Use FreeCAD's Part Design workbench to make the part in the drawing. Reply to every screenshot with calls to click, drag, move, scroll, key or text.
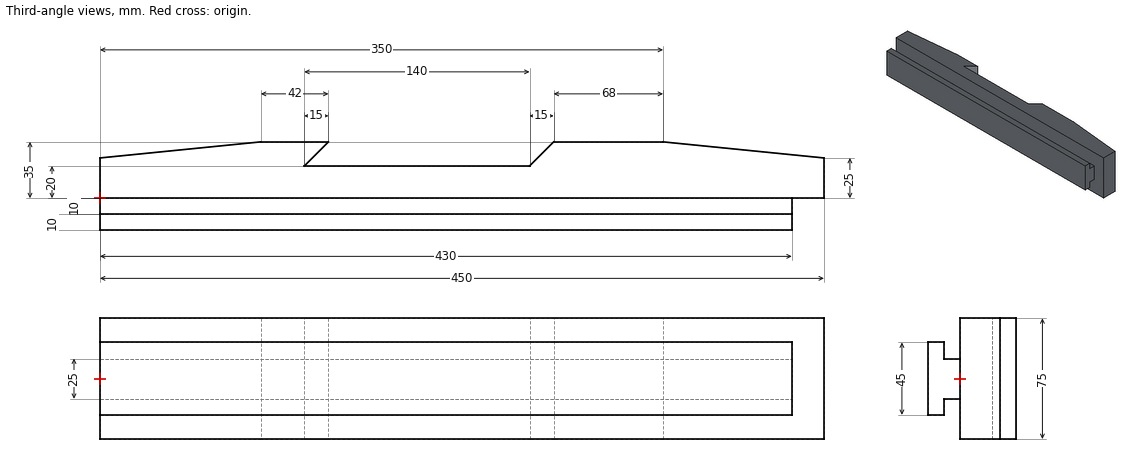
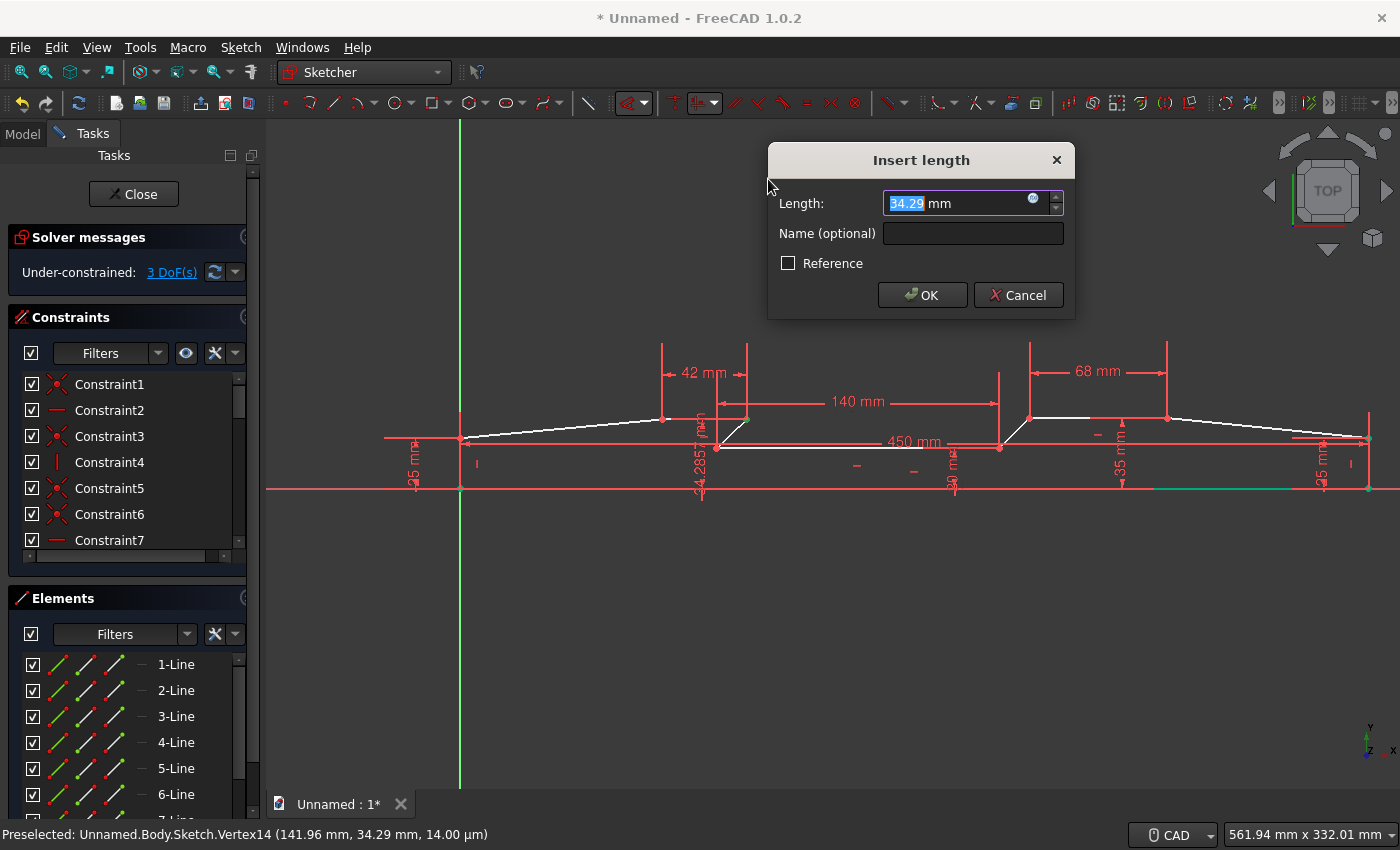
text(35)
key(Return)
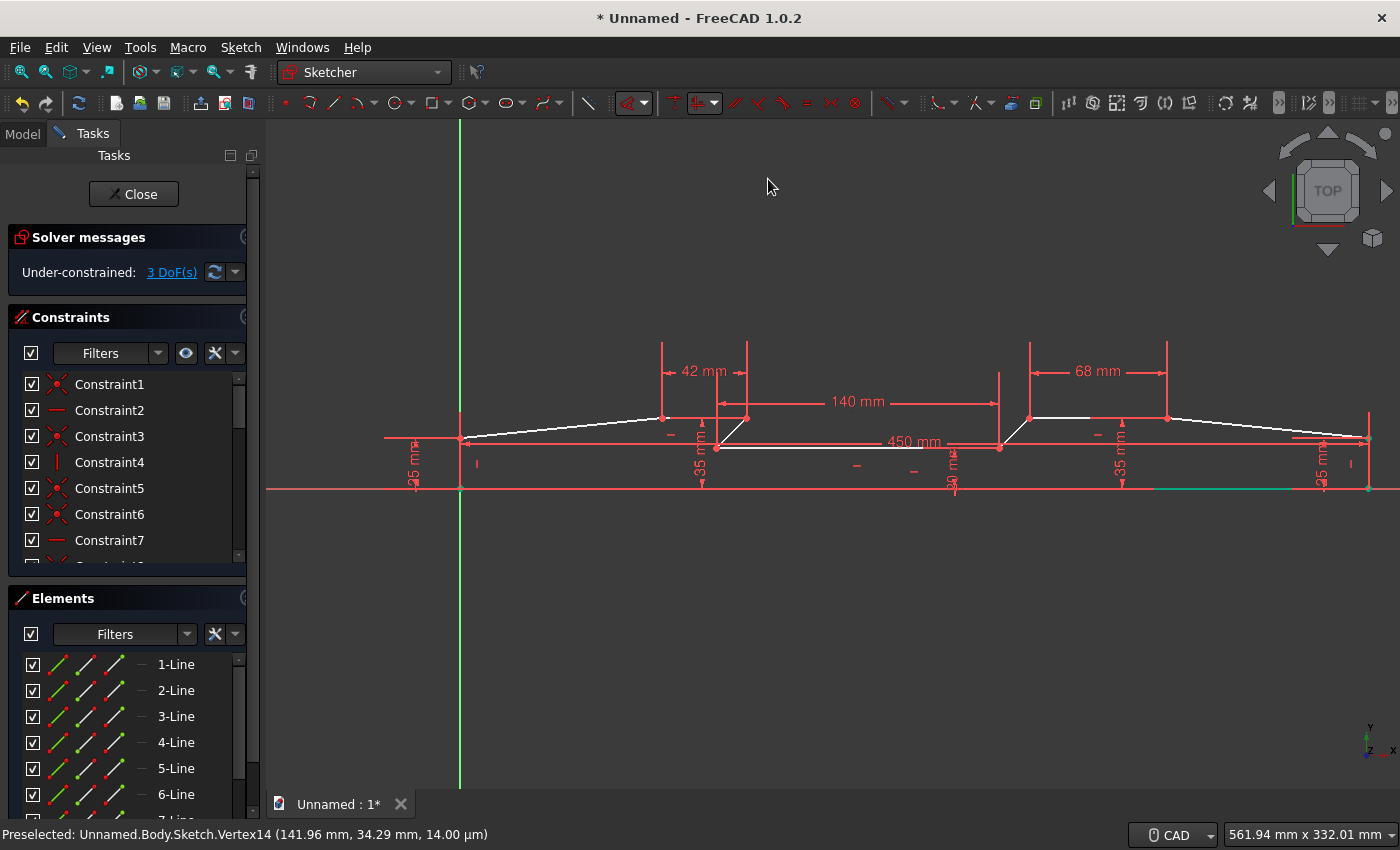
scroll(1021, 427, up, 2)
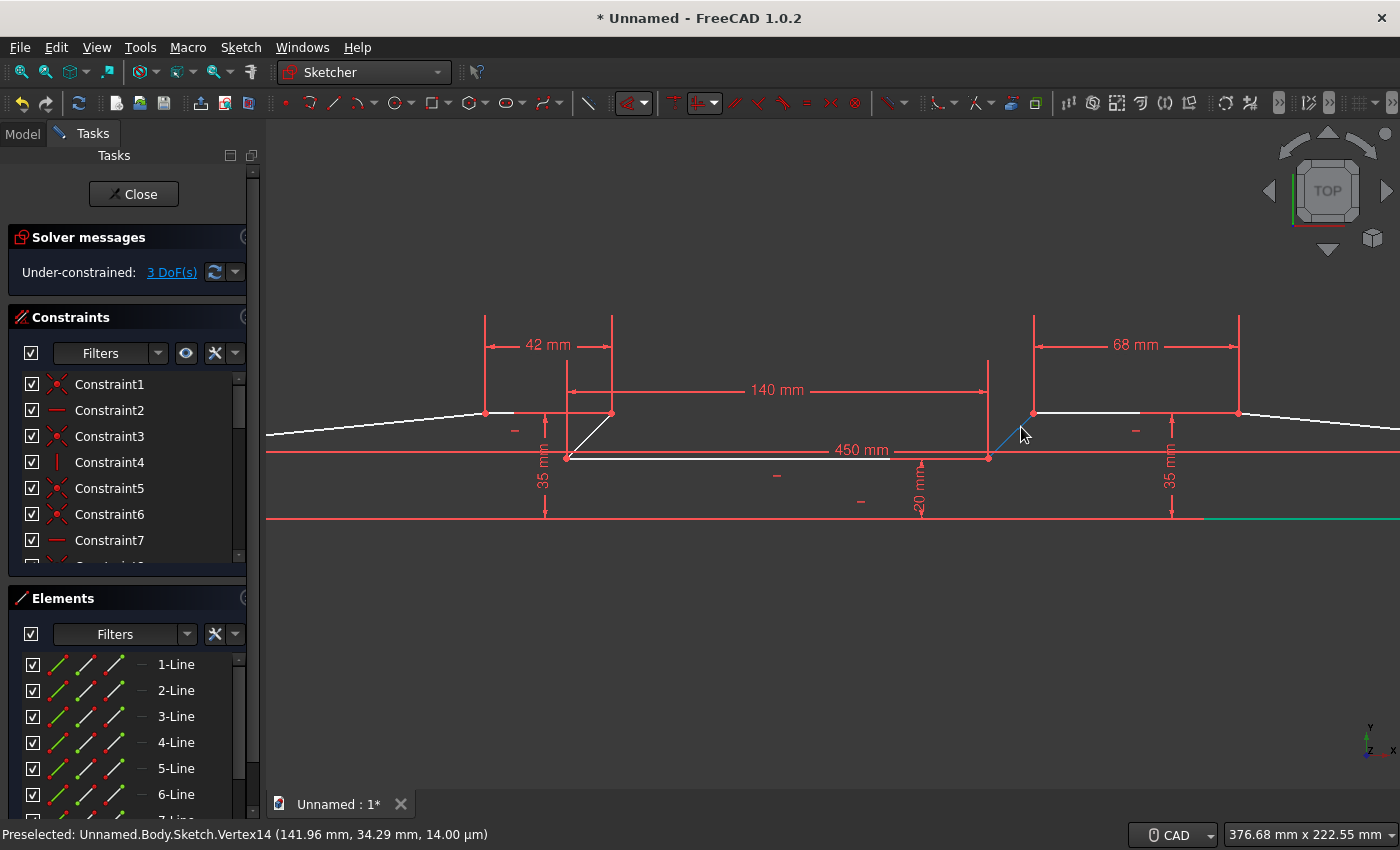
click(1020, 427)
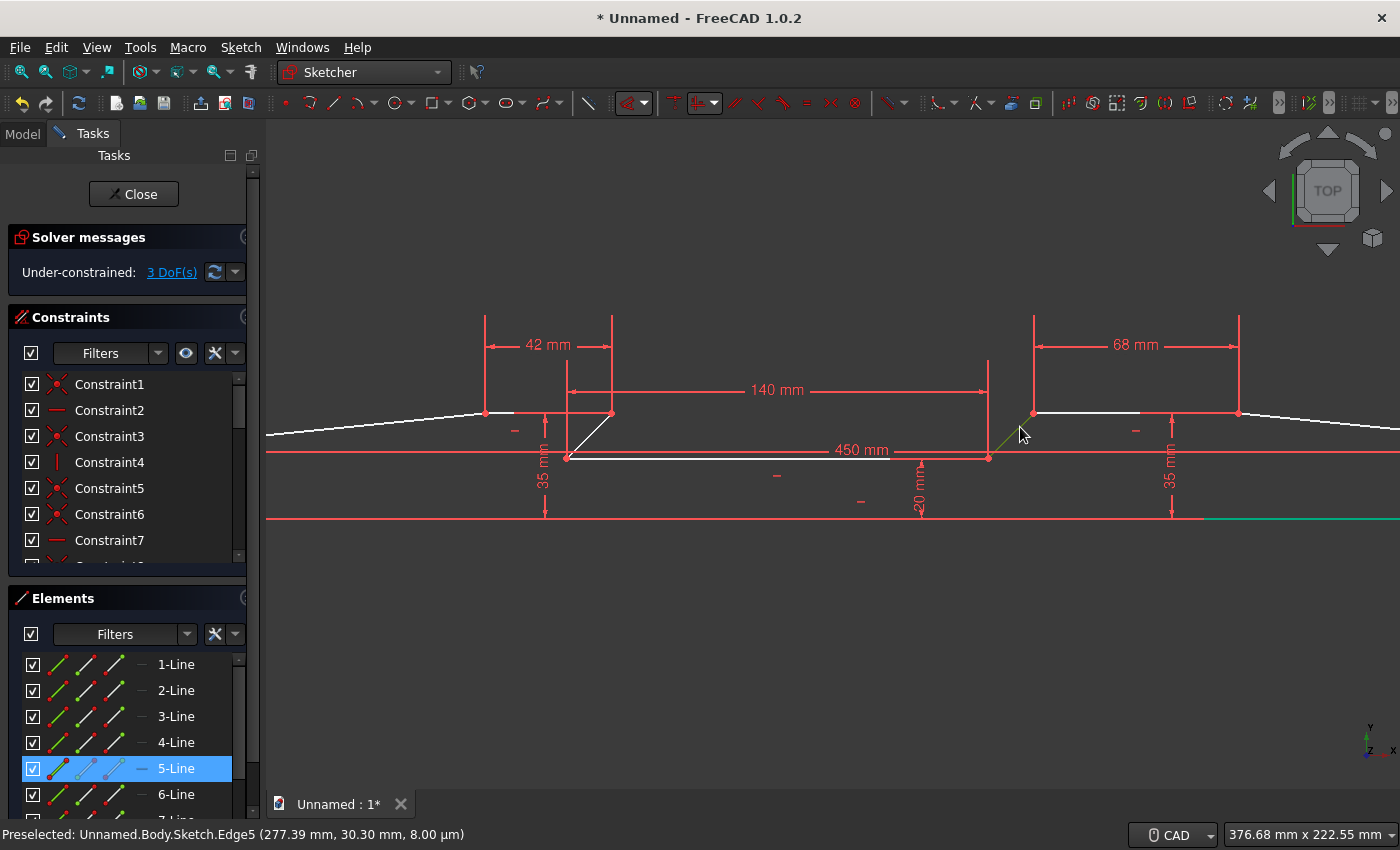
click(646, 104)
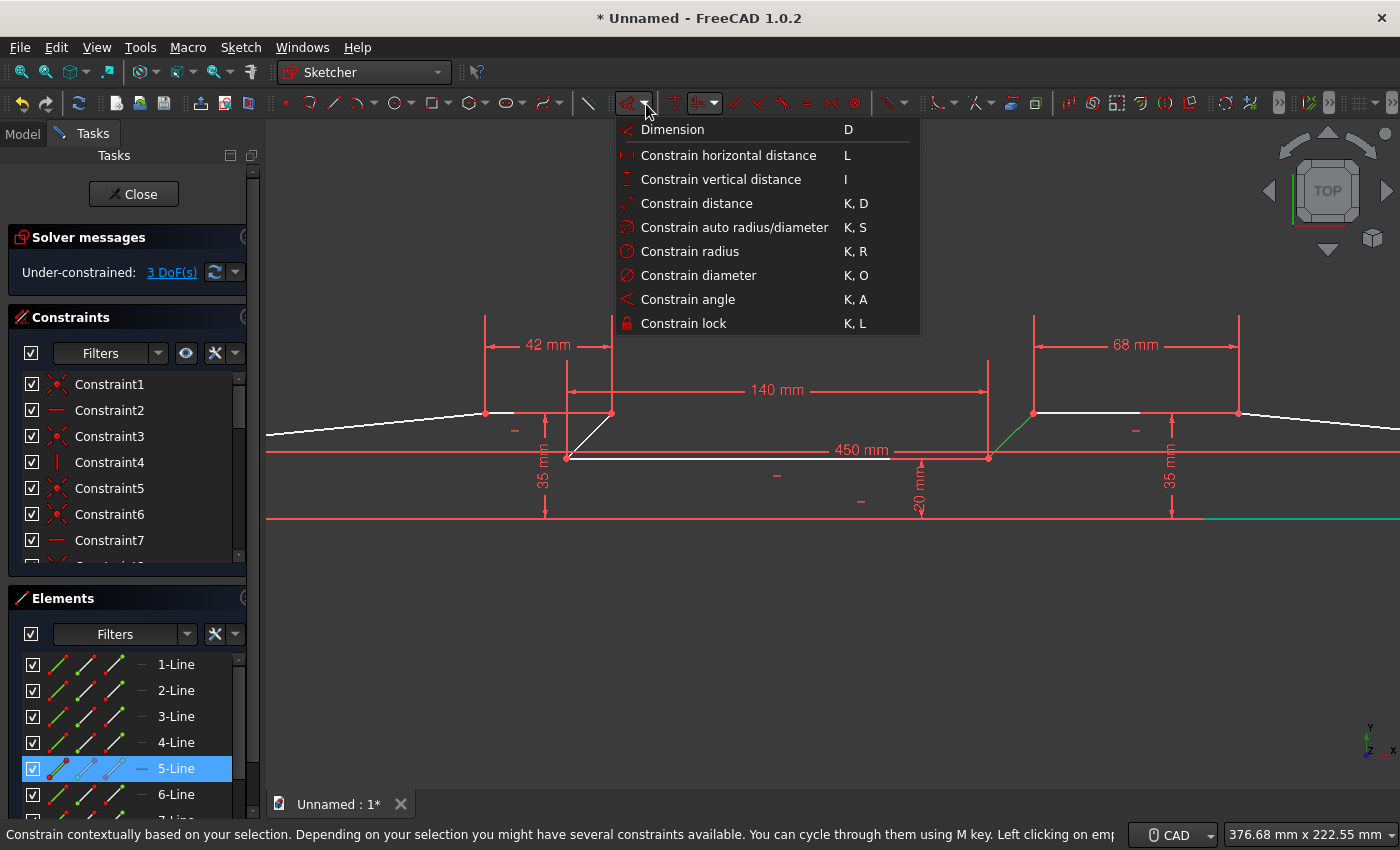
click(768, 155)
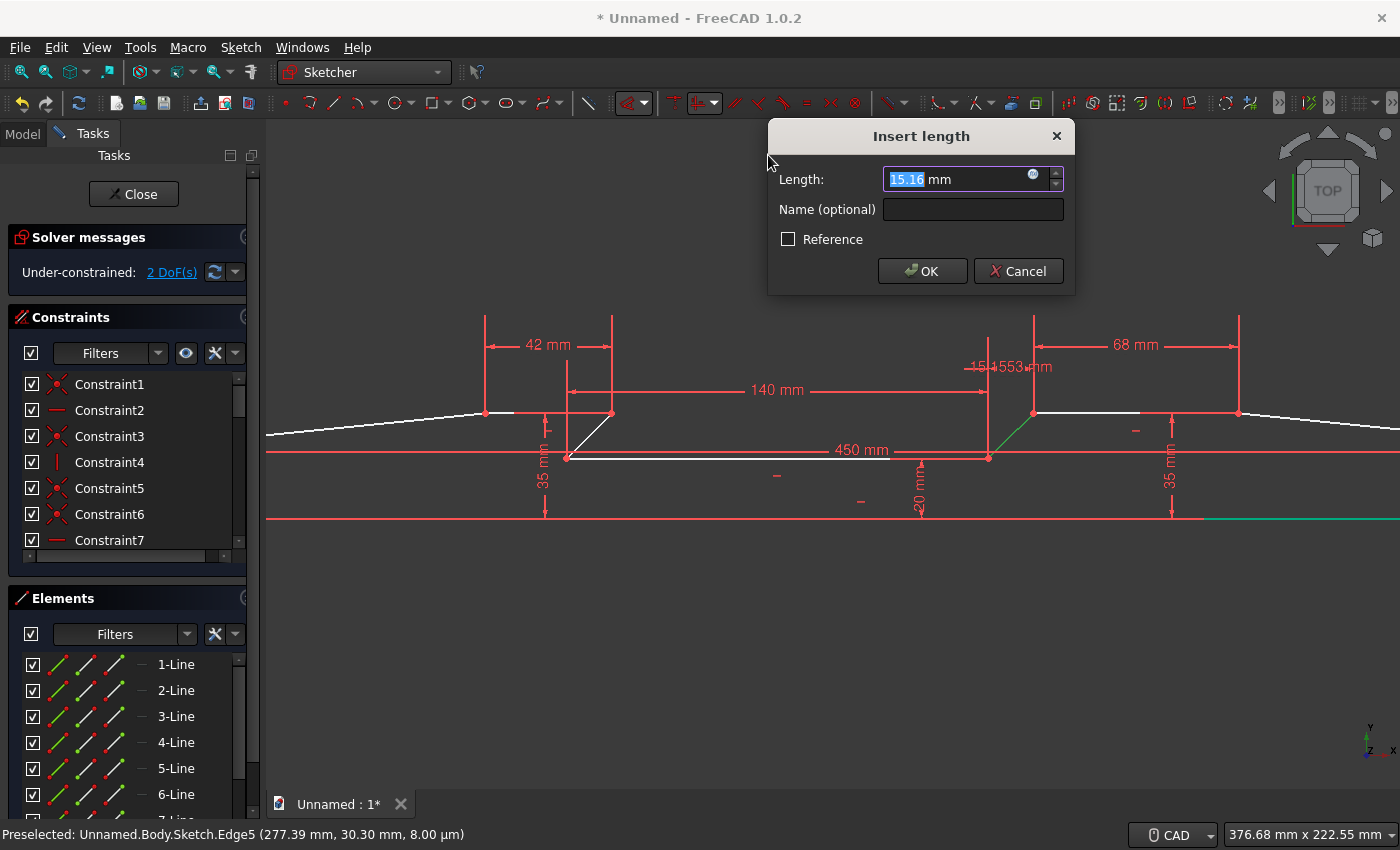
text(15)
key(Return)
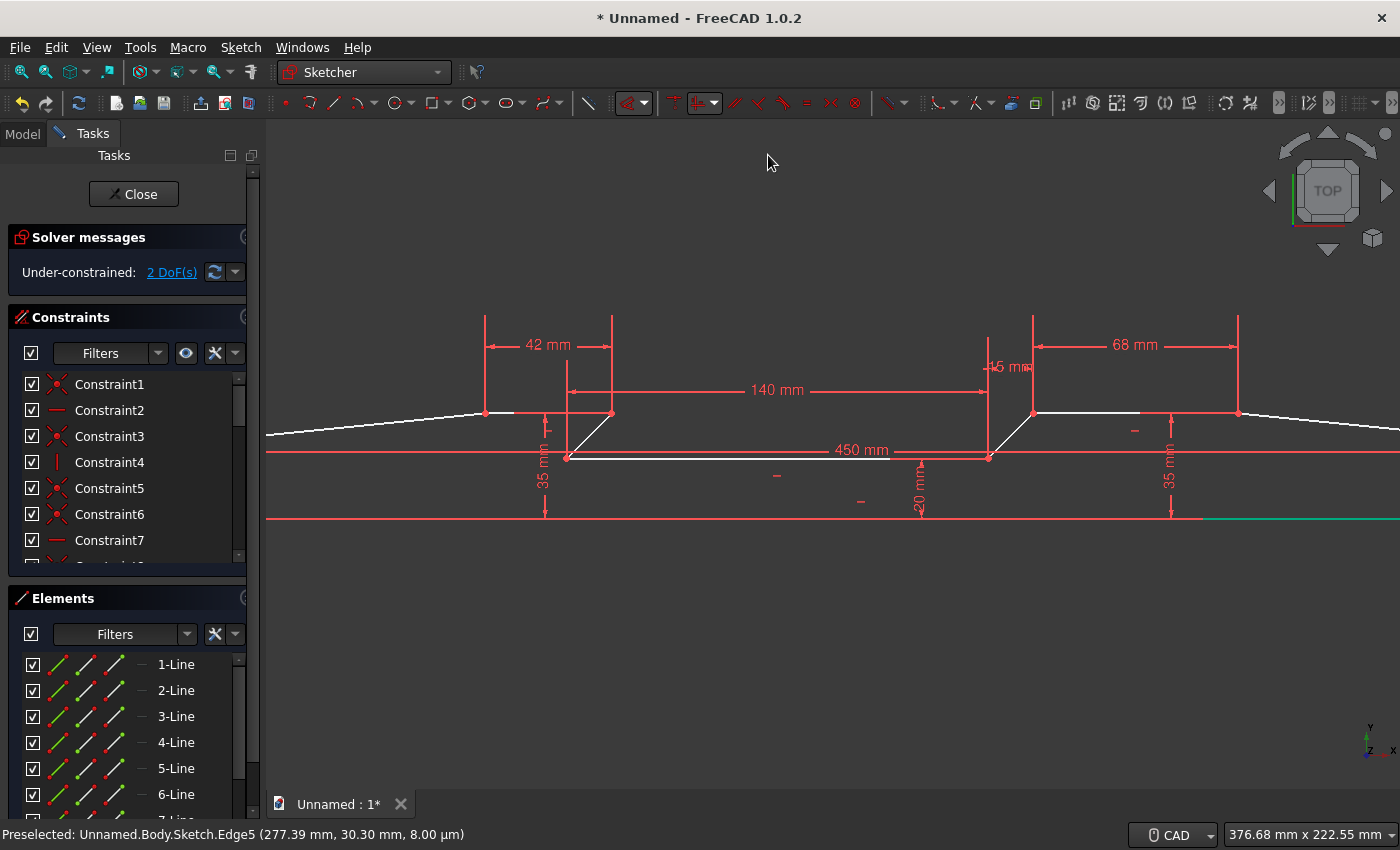
click(580, 445)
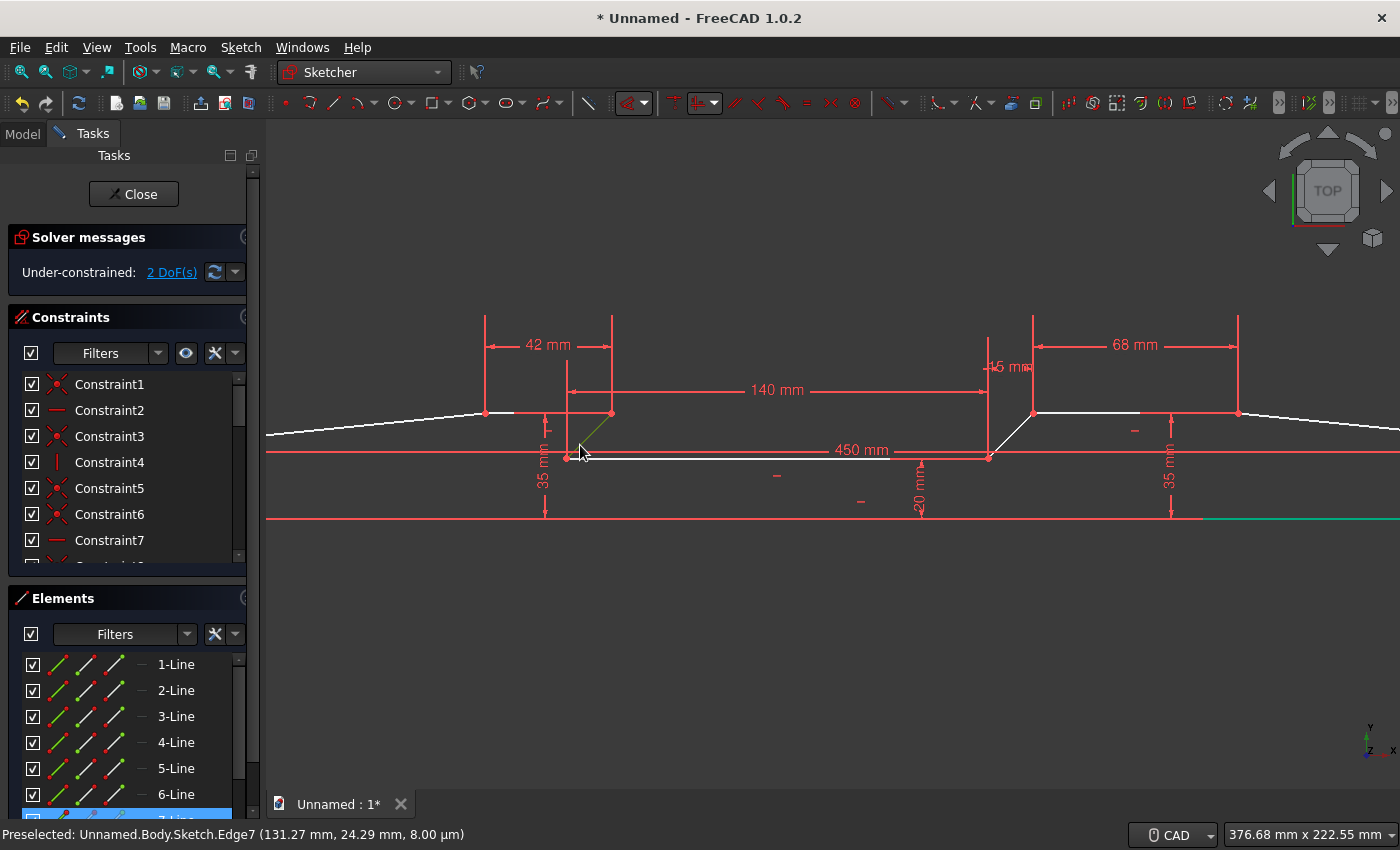
click(646, 104)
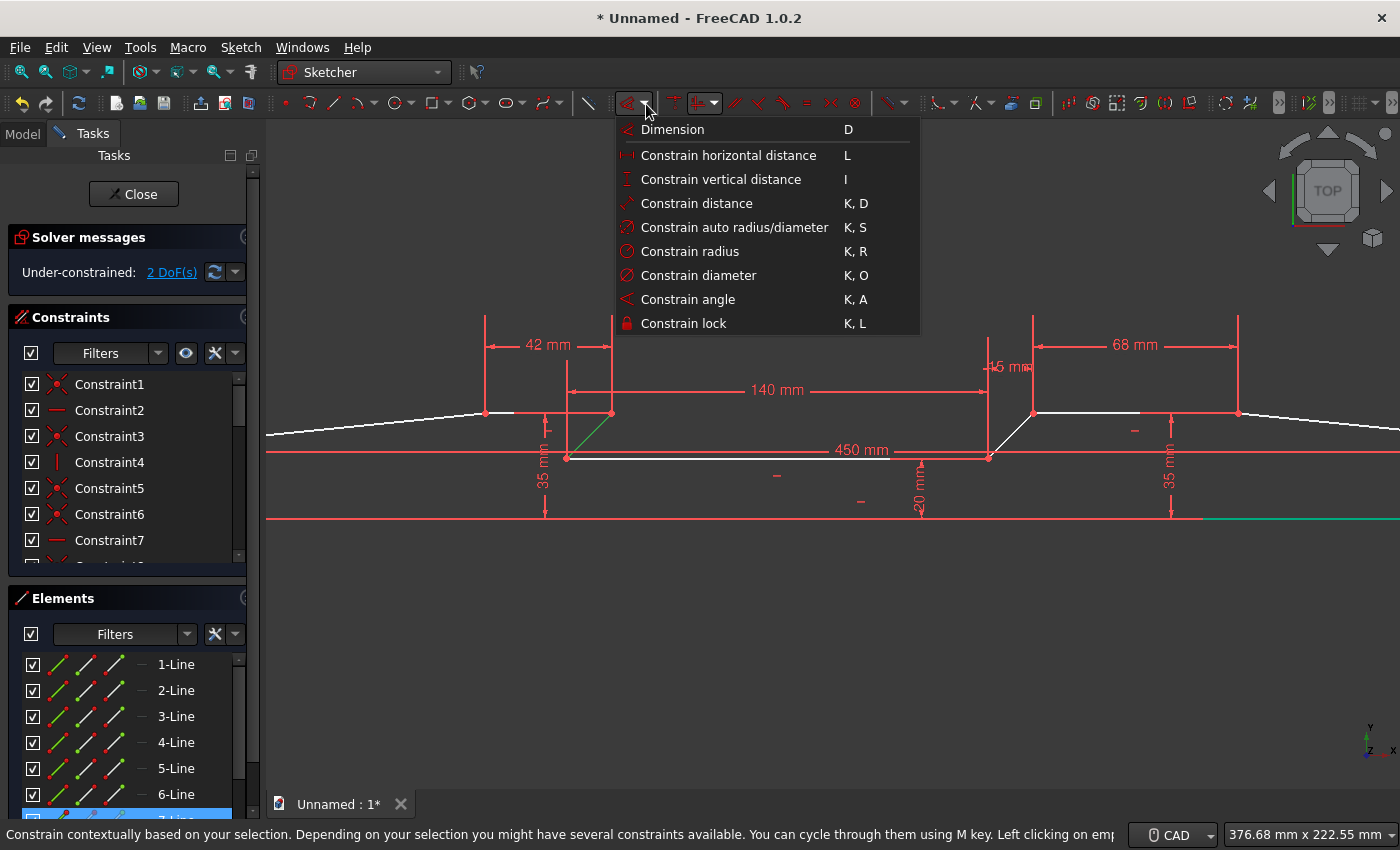
click(768, 155)